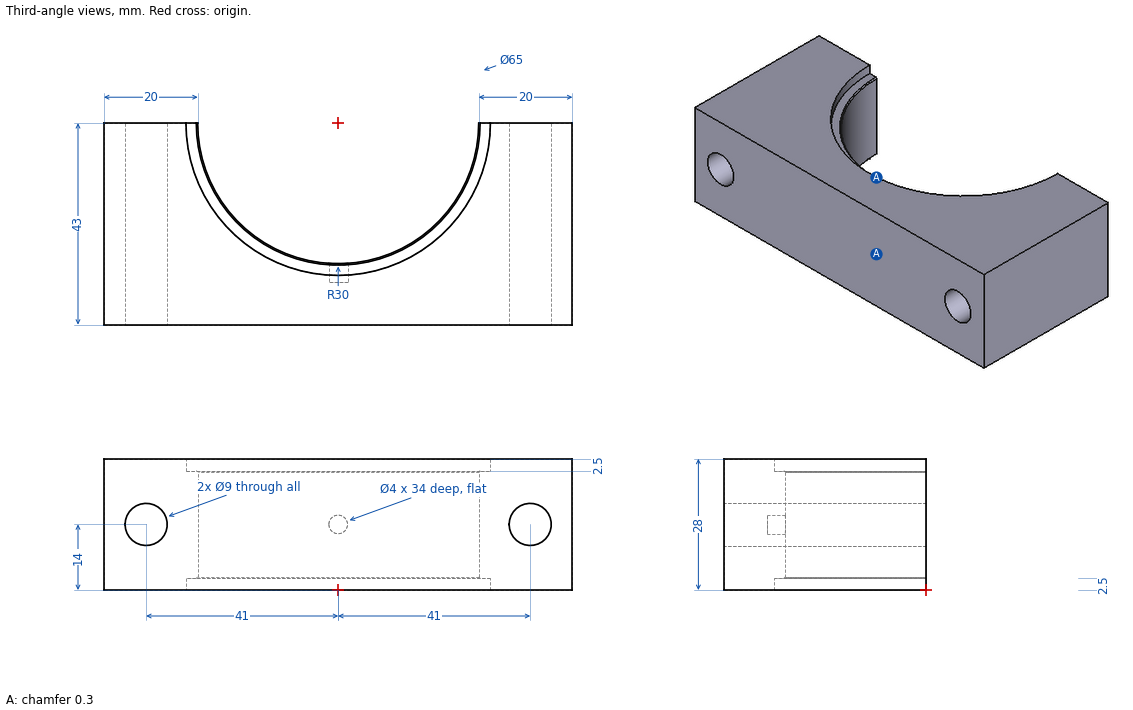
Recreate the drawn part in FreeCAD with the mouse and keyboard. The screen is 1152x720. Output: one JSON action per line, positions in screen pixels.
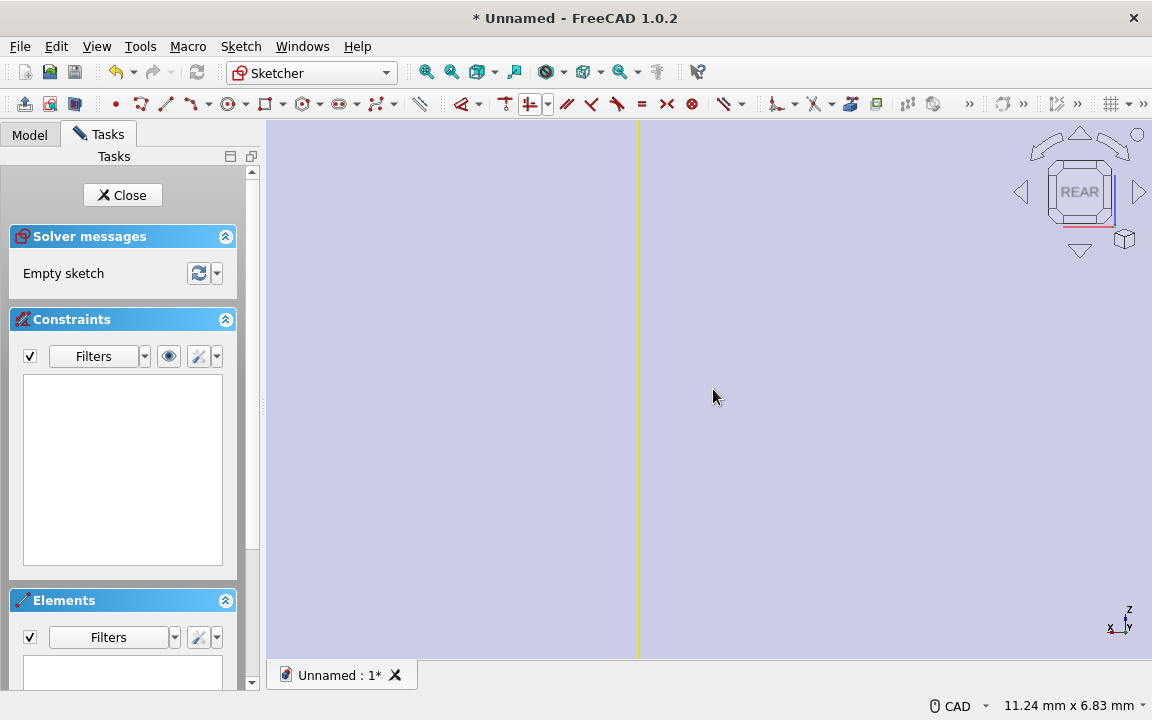
{"action": "left_click", "coordinate": [228, 104]}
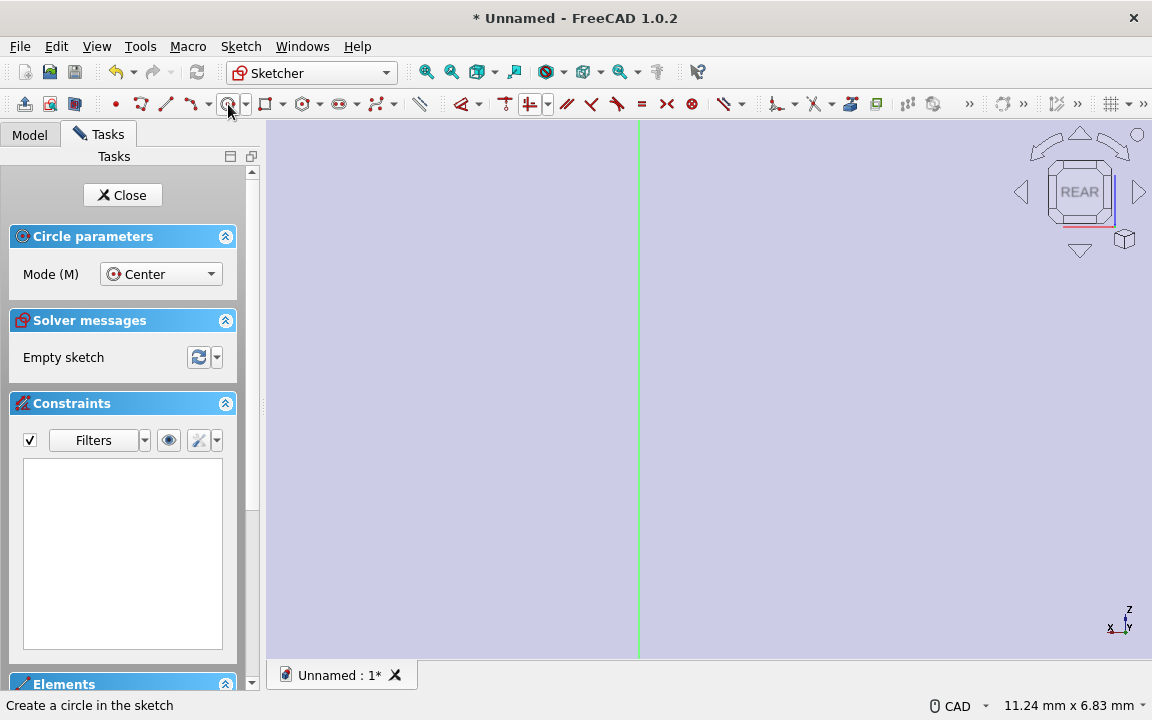
{"action": "left_click", "coordinate": [639, 389]}
{"action": "left_click", "coordinate": [751, 278]}
{"action": "key", "text": "Escape"}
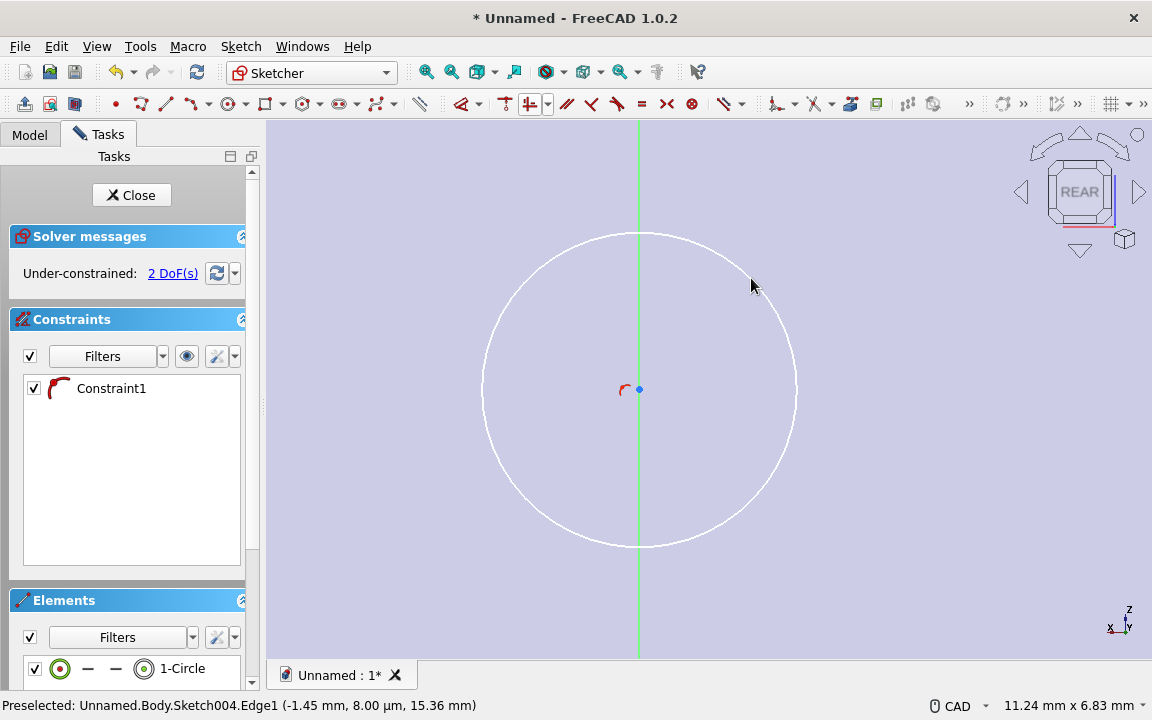
{"action": "left_click", "coordinate": [460, 104]}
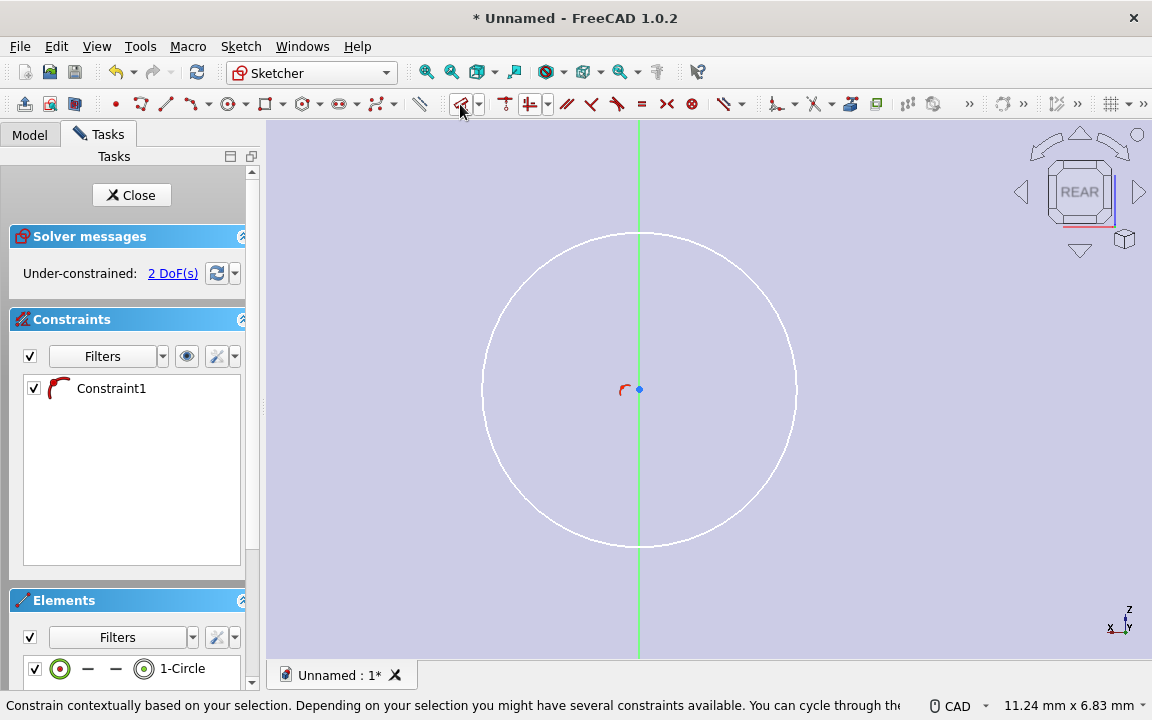
{"action": "left_click", "coordinate": [750, 278]}
{"action": "left_click", "coordinate": [772, 255]}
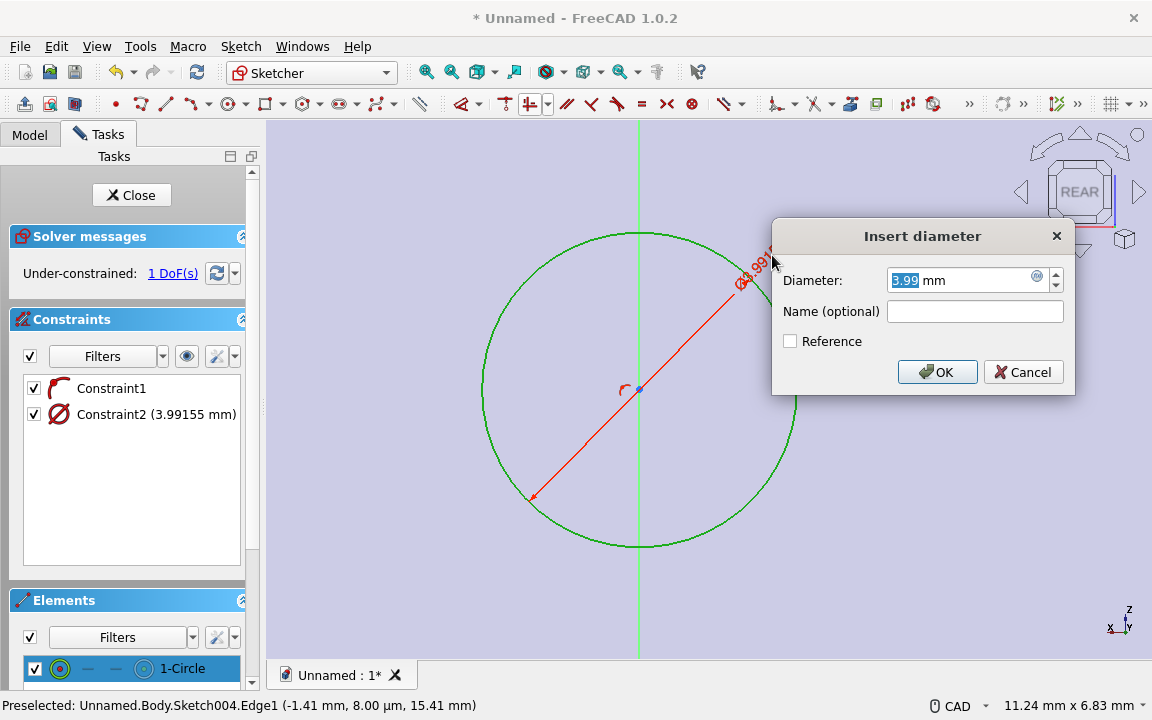
{"action": "type", "text": "4"}
{"action": "key", "text": "Return"}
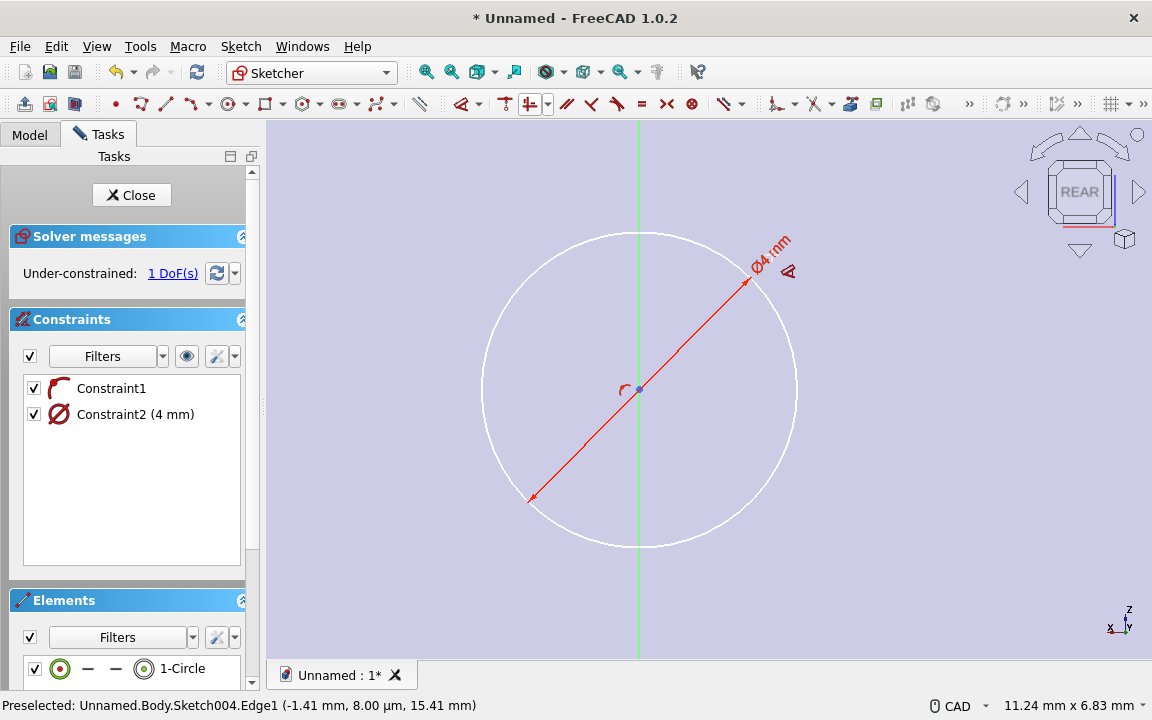
{"action": "left_click", "coordinate": [639, 390]}
{"action": "left_click", "coordinate": [673, 510]}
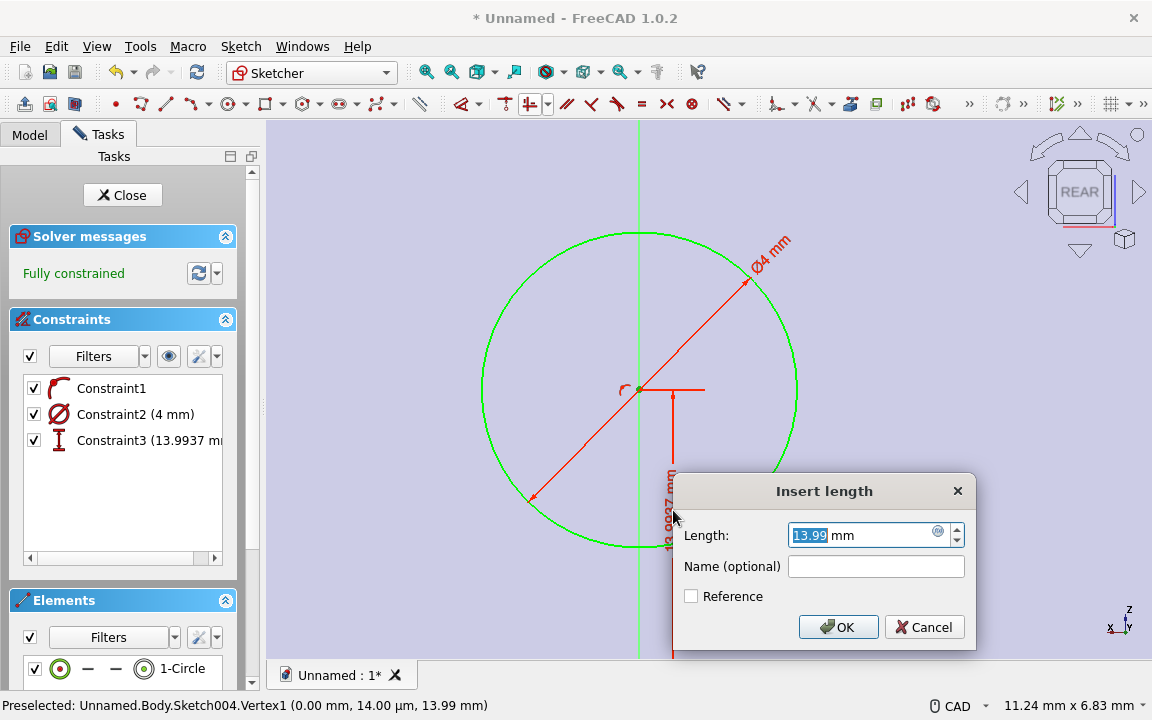
{"action": "type", "text": "14"}
{"action": "key", "text": "Return"}
{"action": "key", "text": "Escape"}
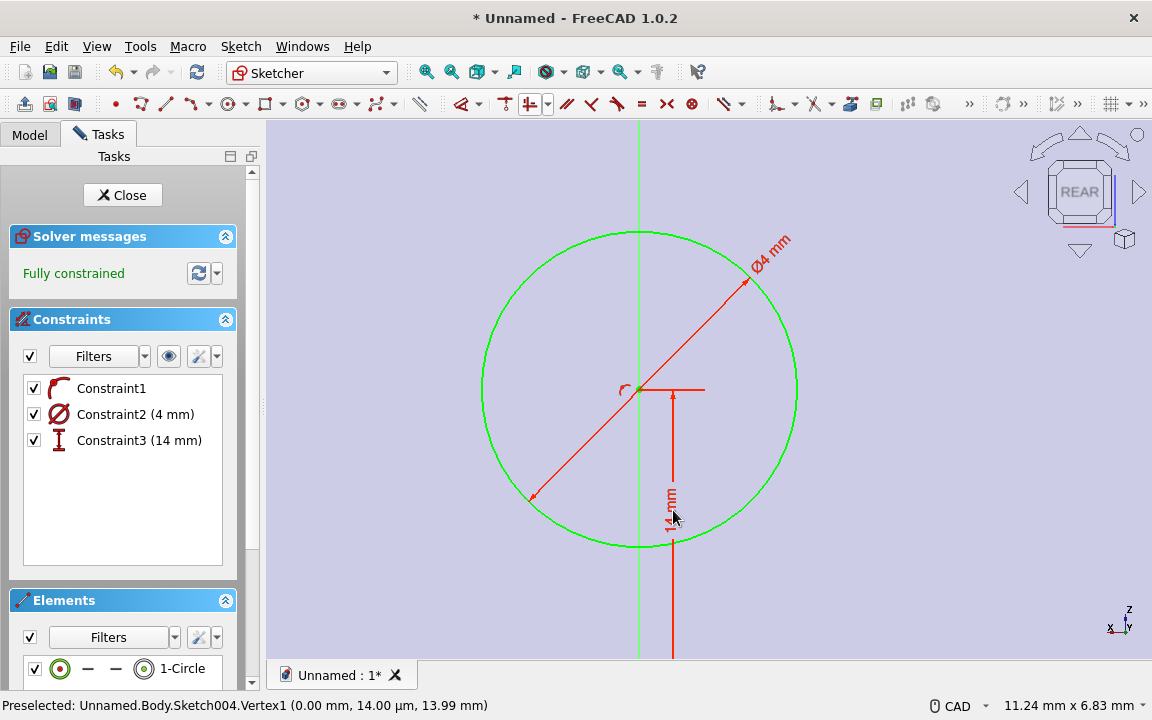
{"action": "left_click", "coordinate": [123, 195]}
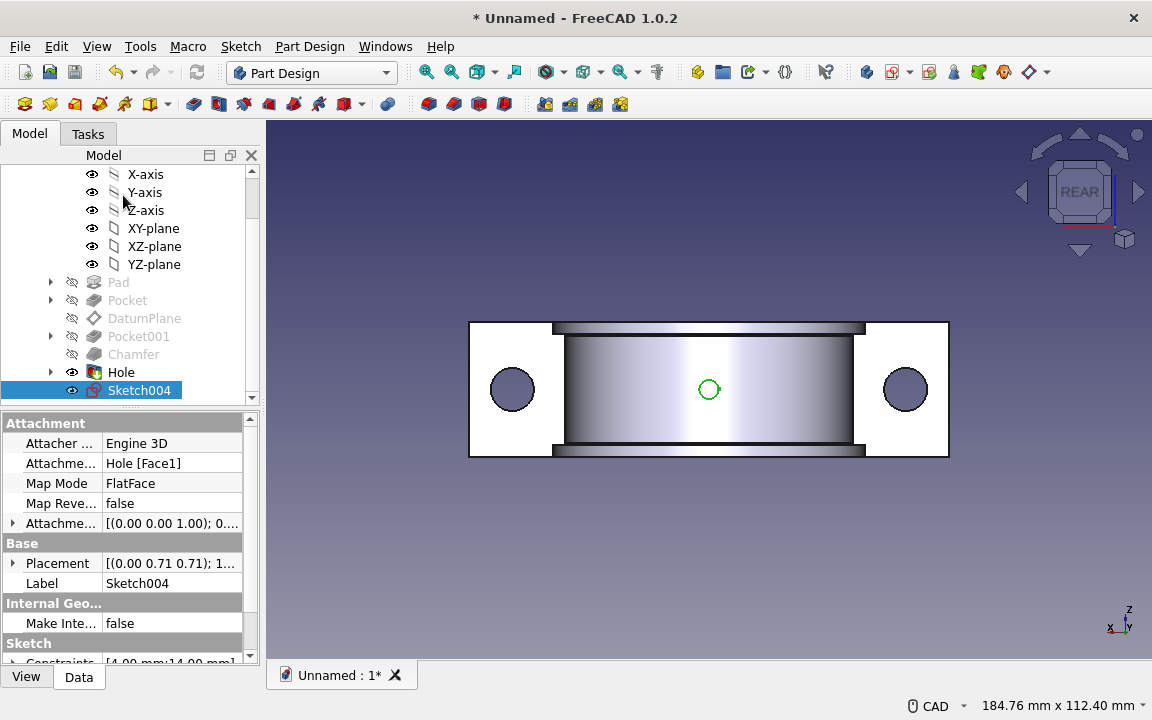
{"action": "left_click", "coordinate": [219, 104]}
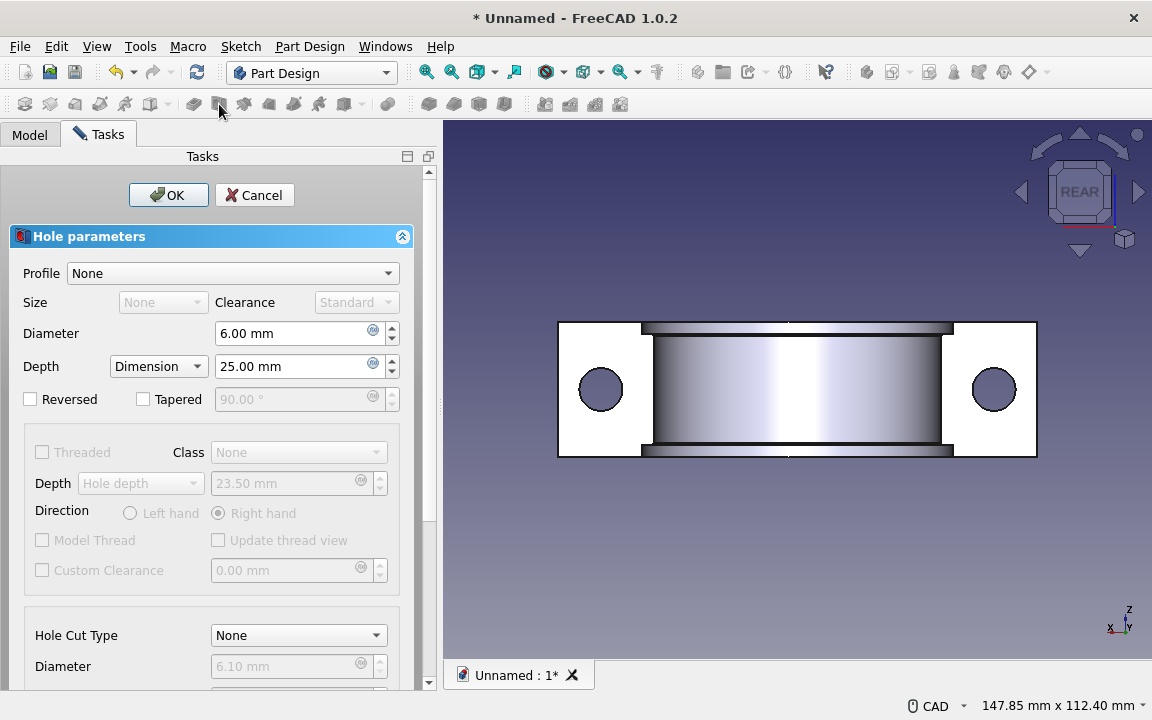
{"action": "triple_click", "coordinate": [300, 334]}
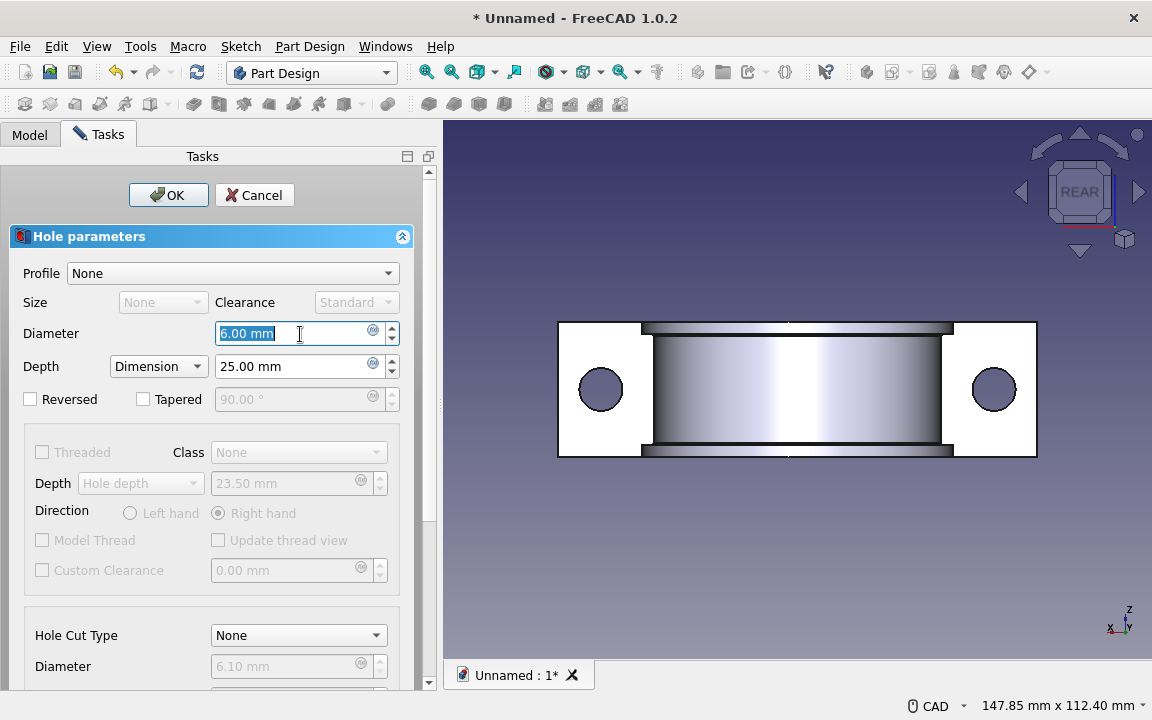
{"action": "type", "text": "4"}
{"action": "key", "text": "Tab"}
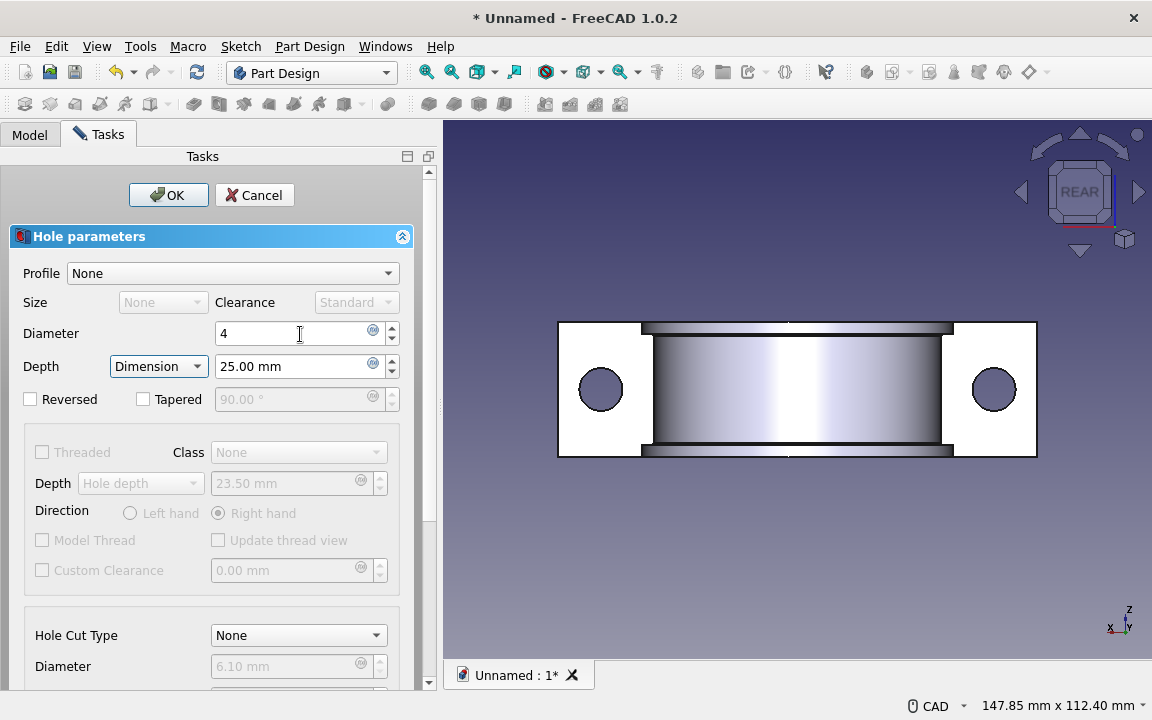
{"action": "triple_click", "coordinate": [300, 366]}